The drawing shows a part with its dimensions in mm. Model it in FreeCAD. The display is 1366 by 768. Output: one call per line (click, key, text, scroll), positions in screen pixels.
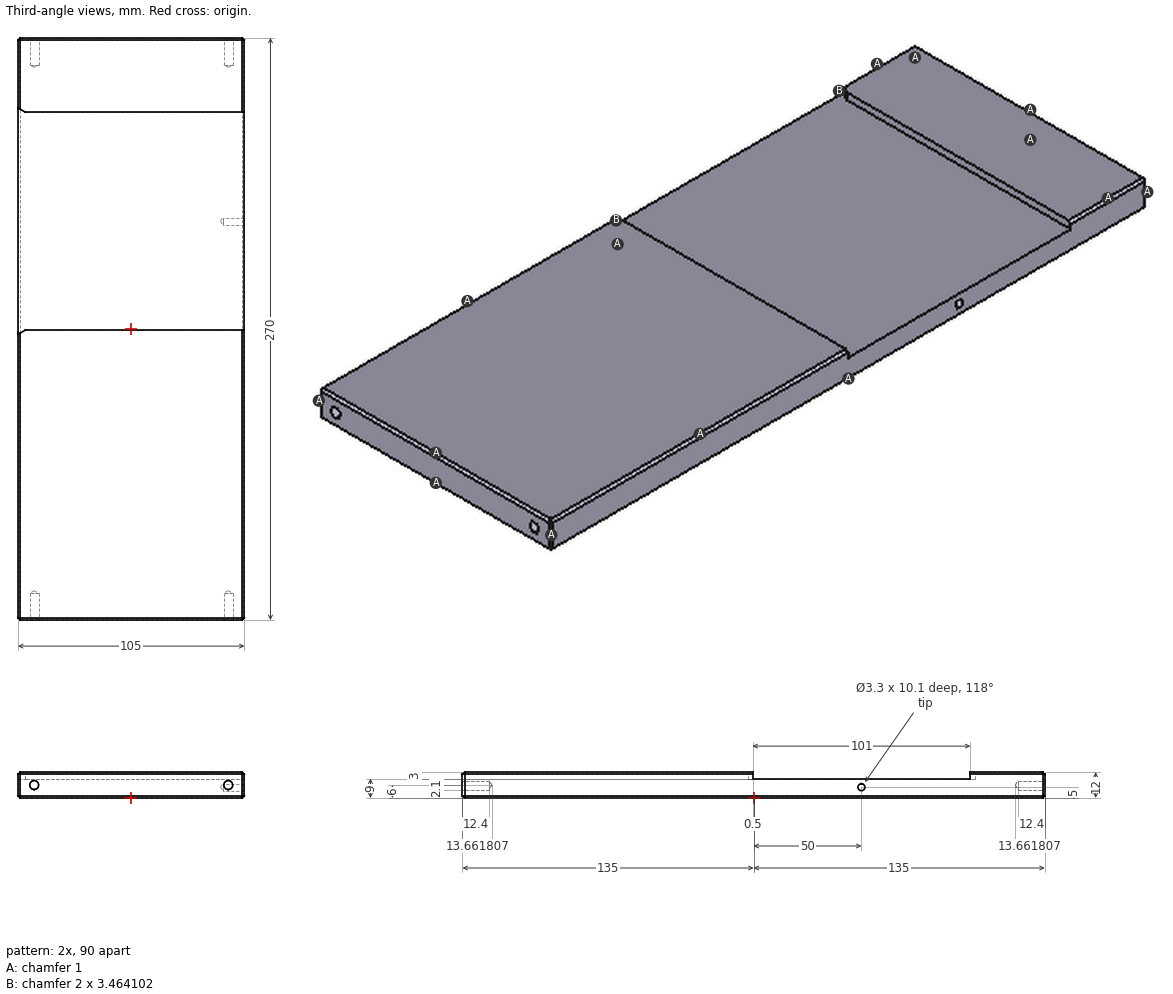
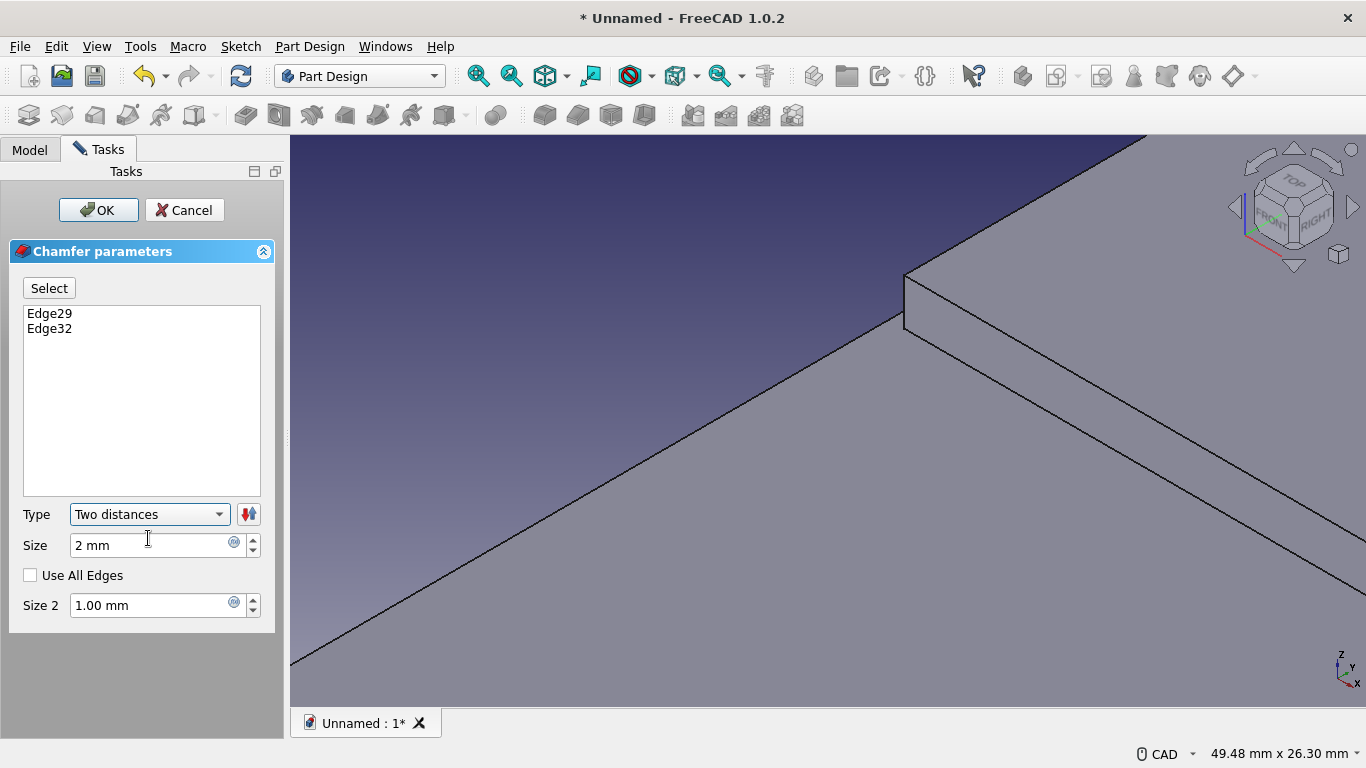
triple_click(158, 606)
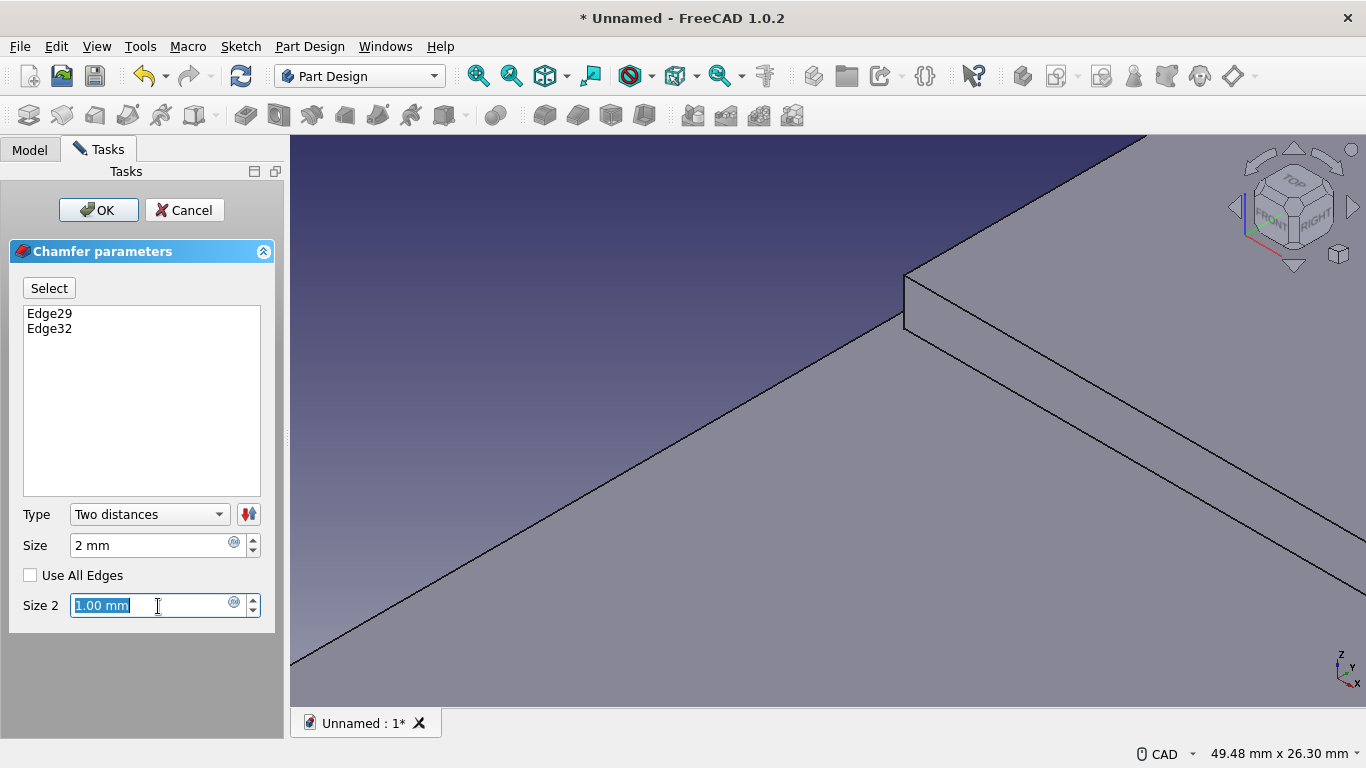
text(3.464102)
key(Tab)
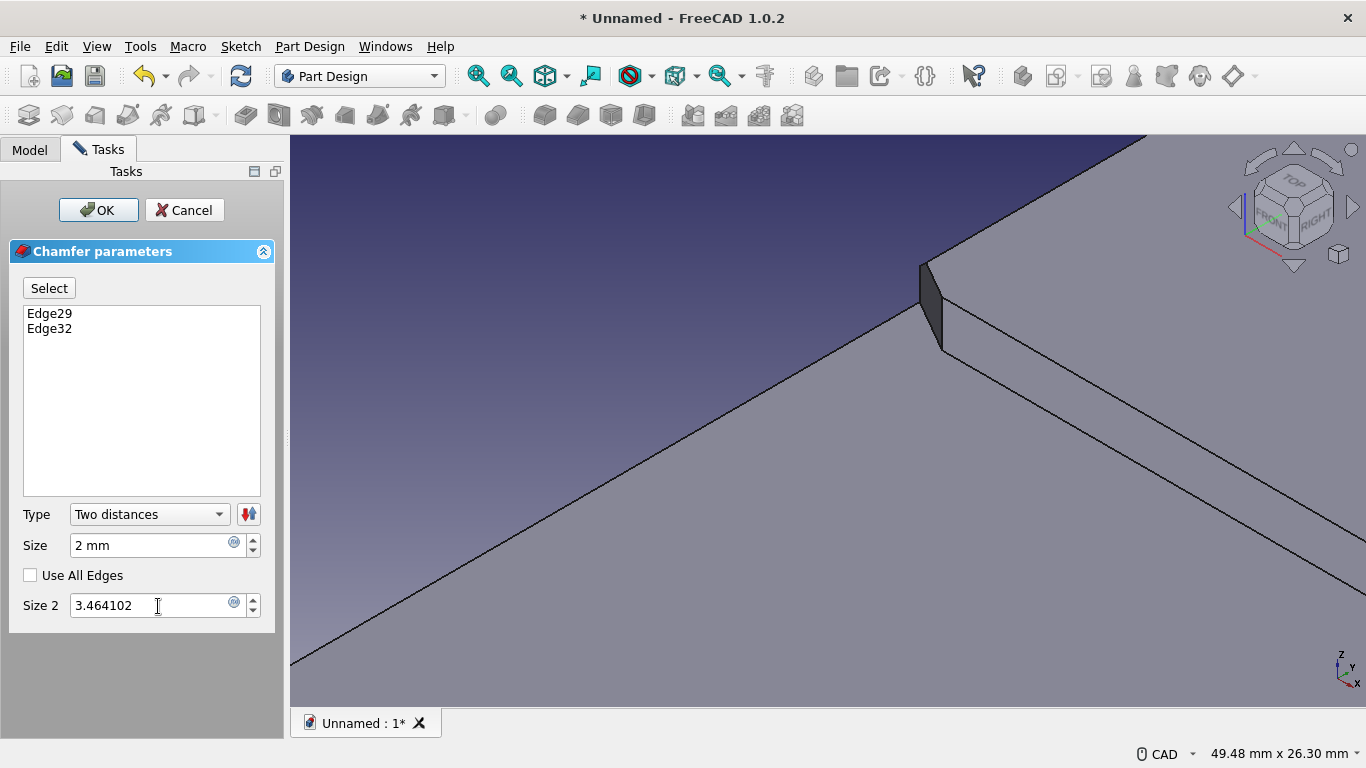
click(99, 210)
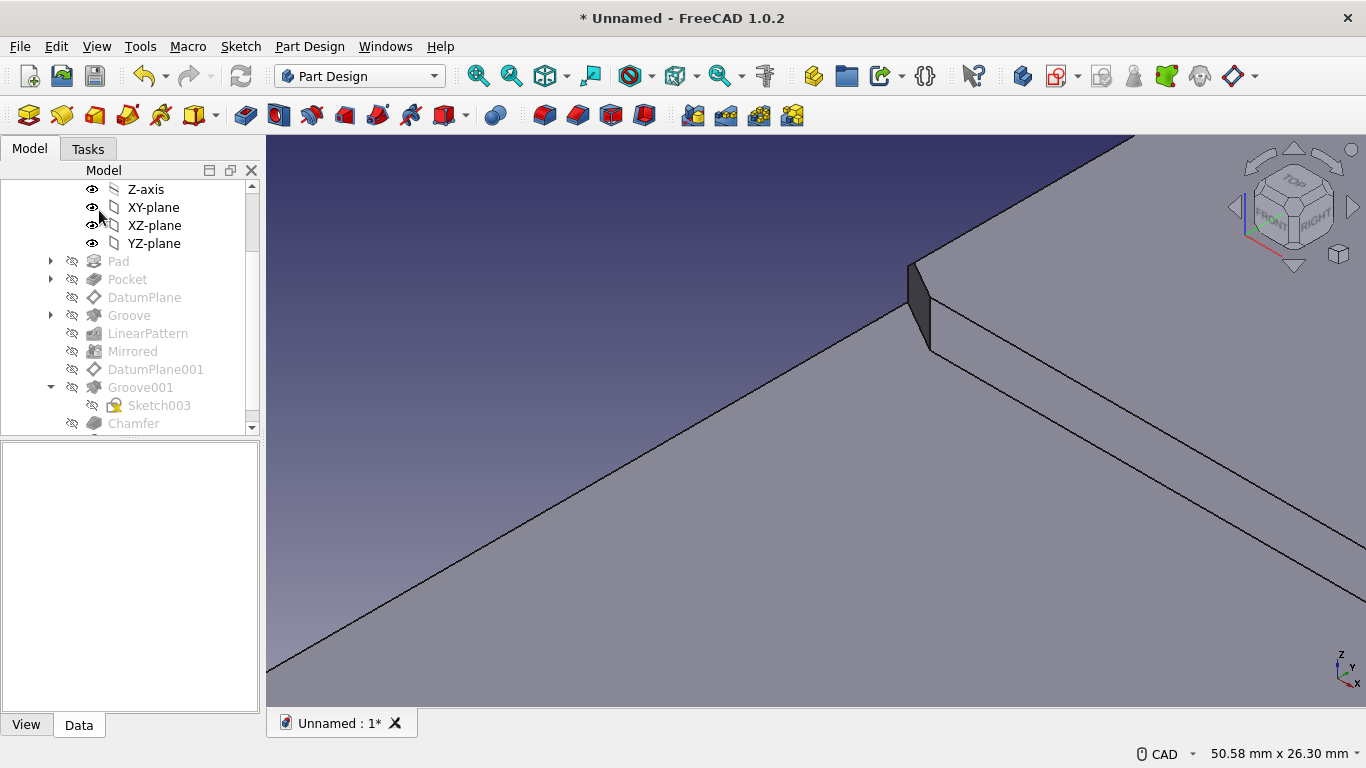
click(479, 76)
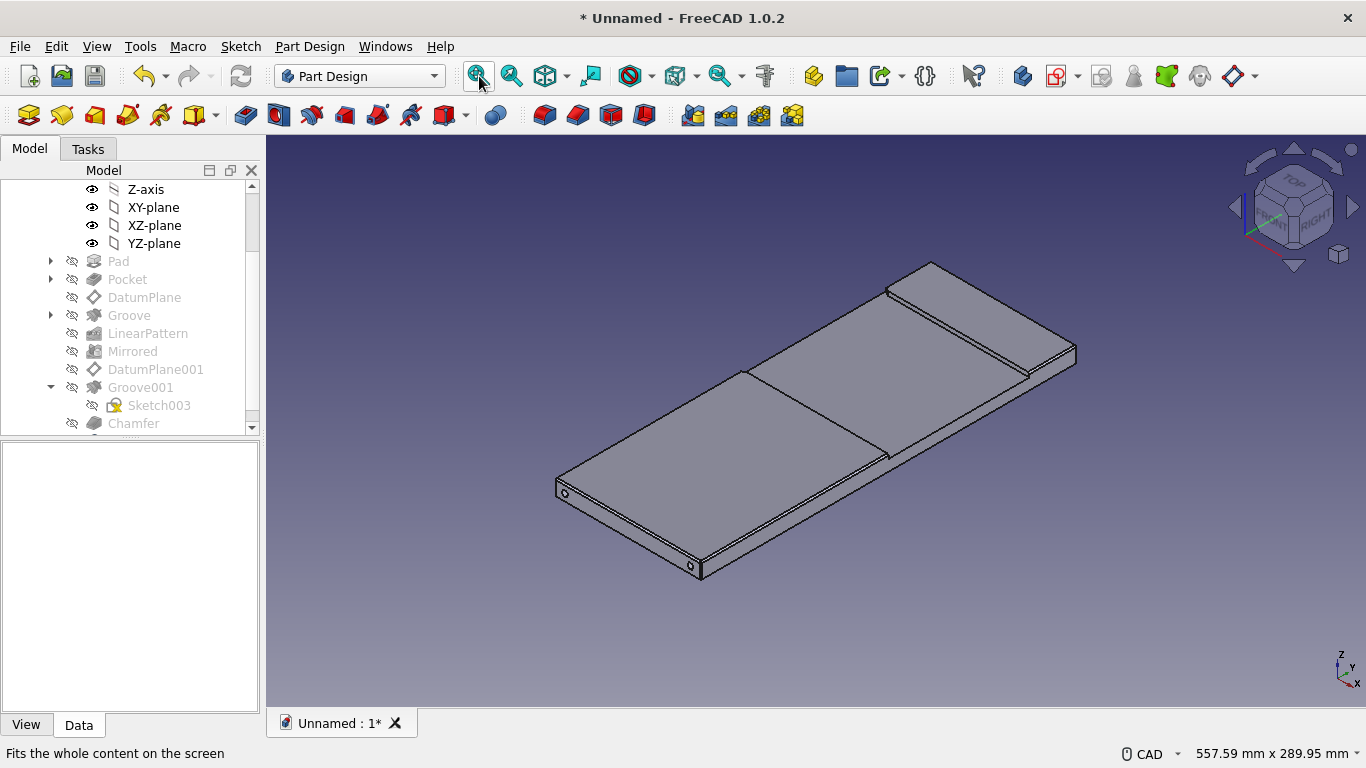
key(3)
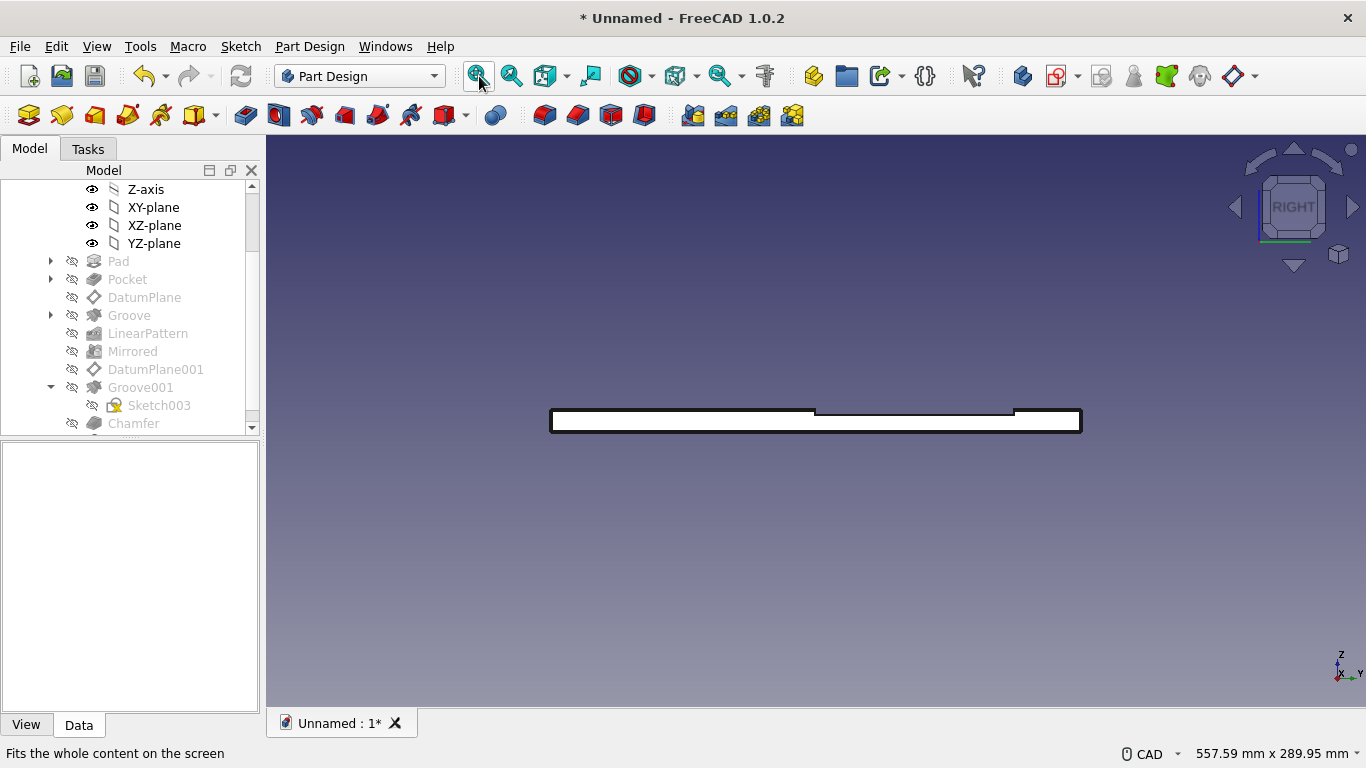
click(1043, 420)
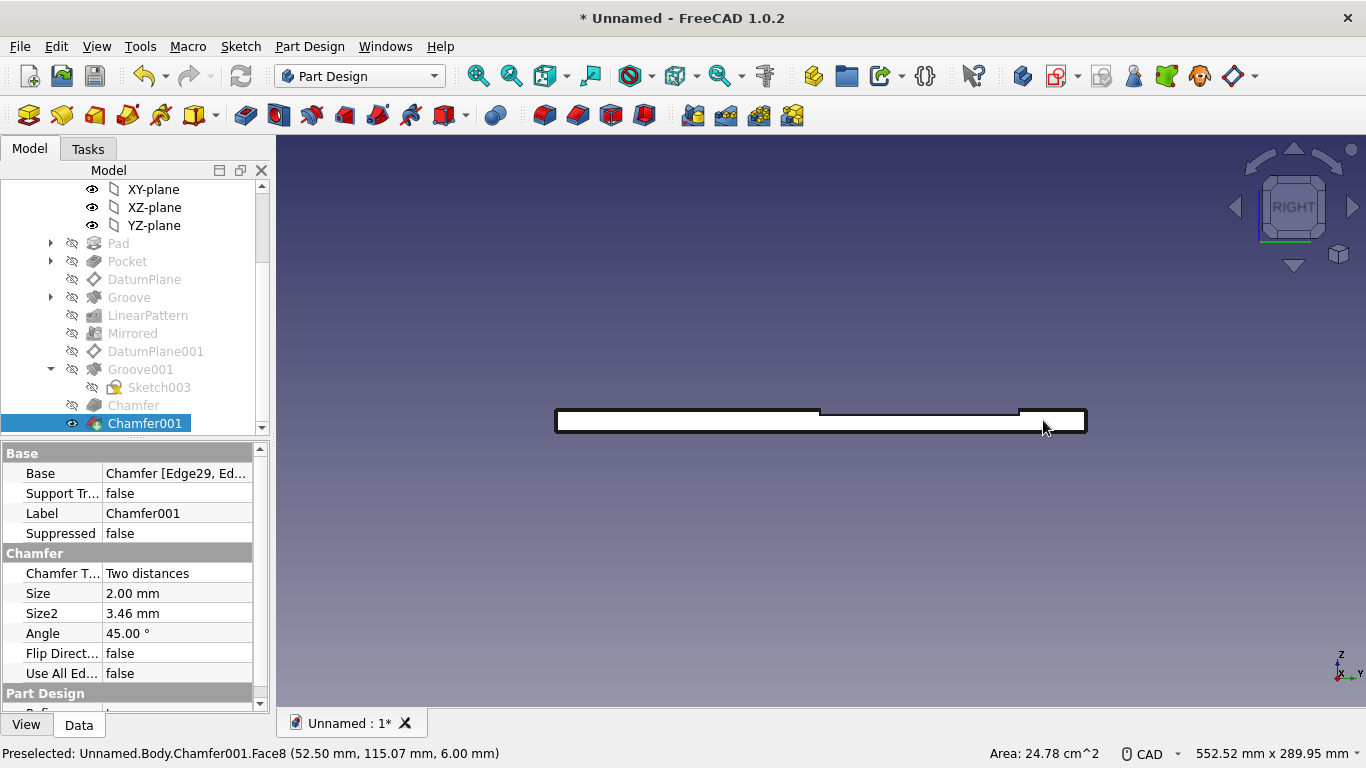
click(1056, 76)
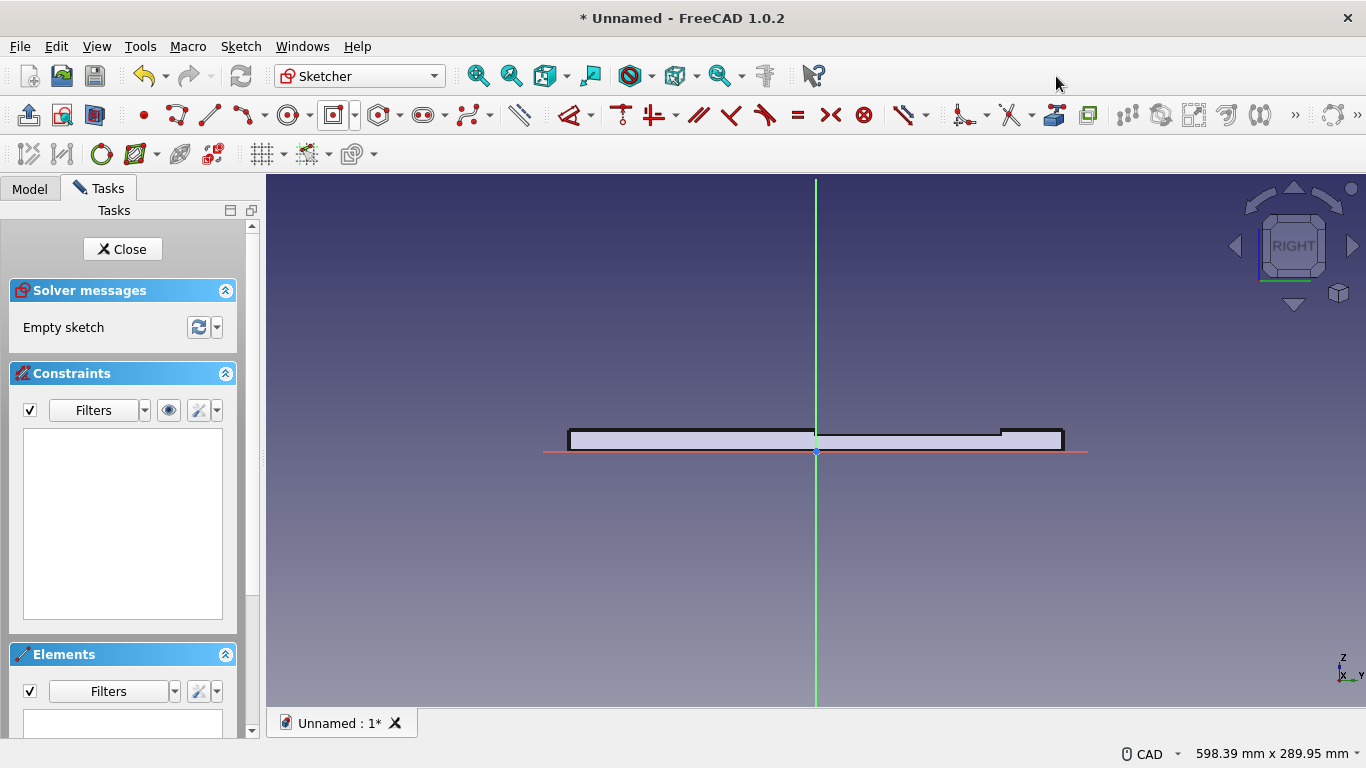
scroll(916, 442, up, 15)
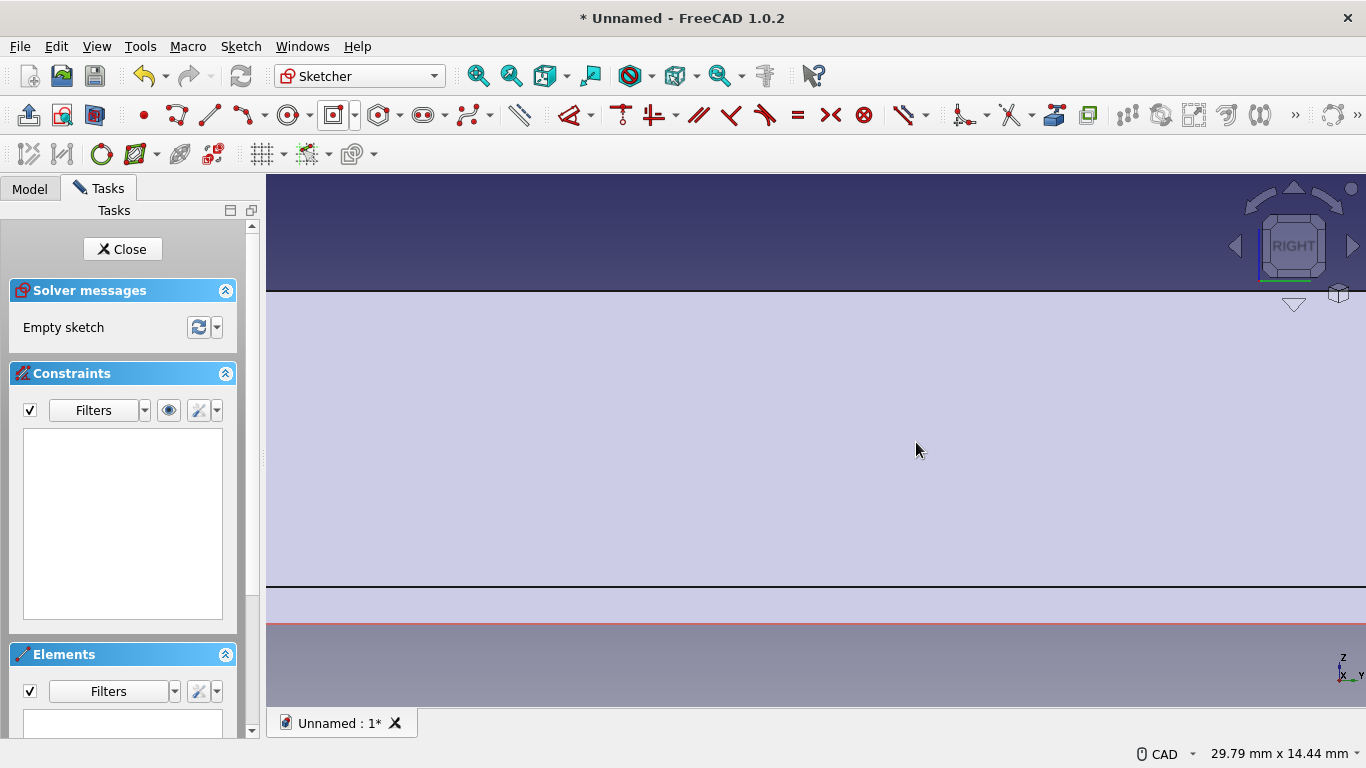
scroll(739, 438, up, 5)